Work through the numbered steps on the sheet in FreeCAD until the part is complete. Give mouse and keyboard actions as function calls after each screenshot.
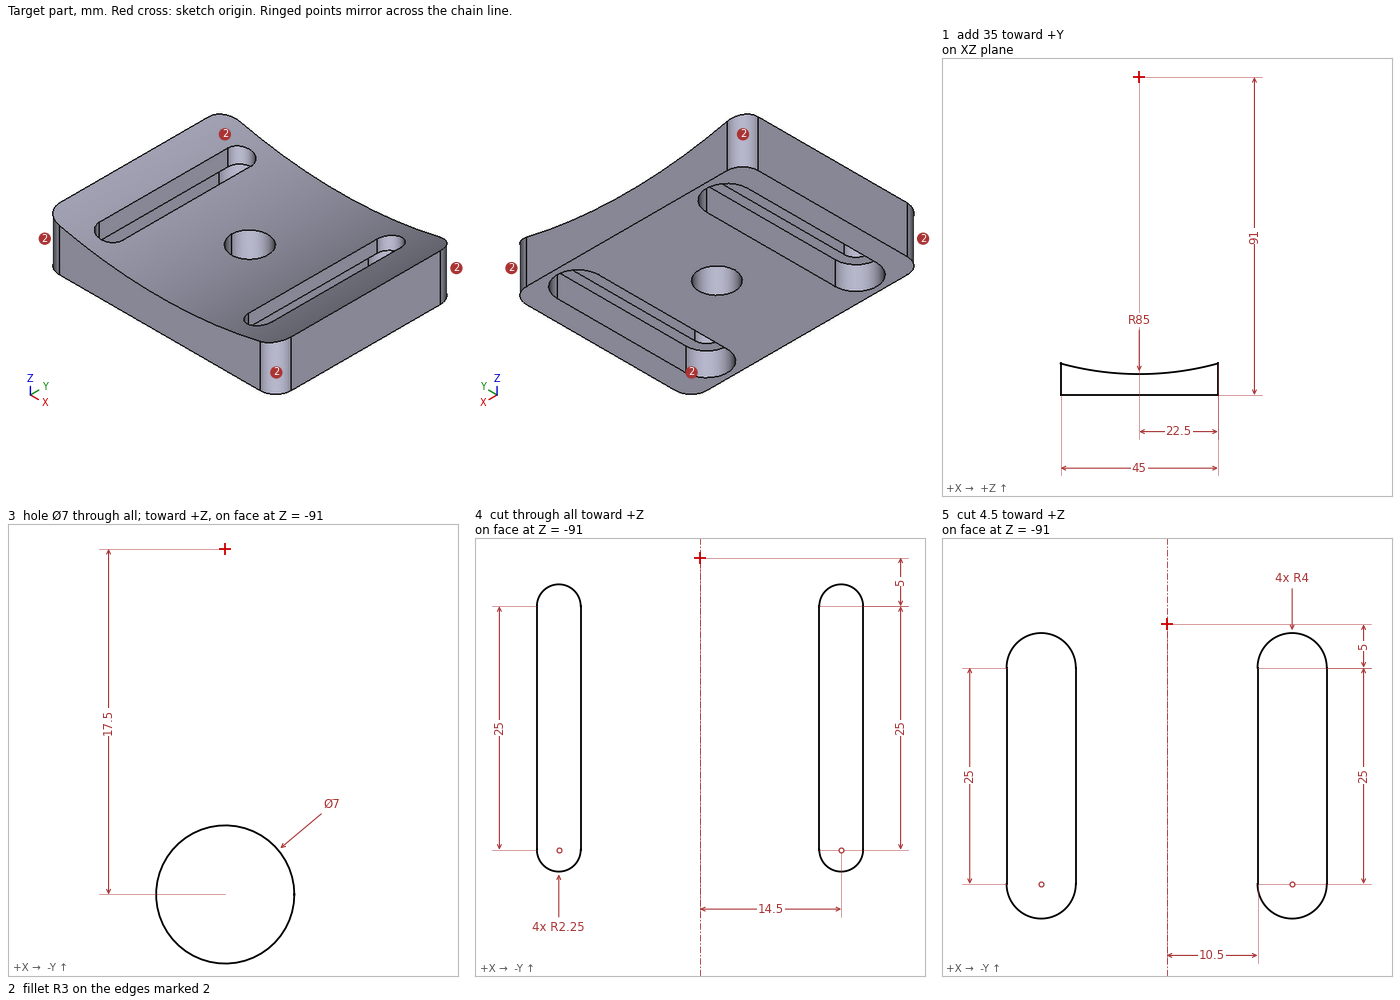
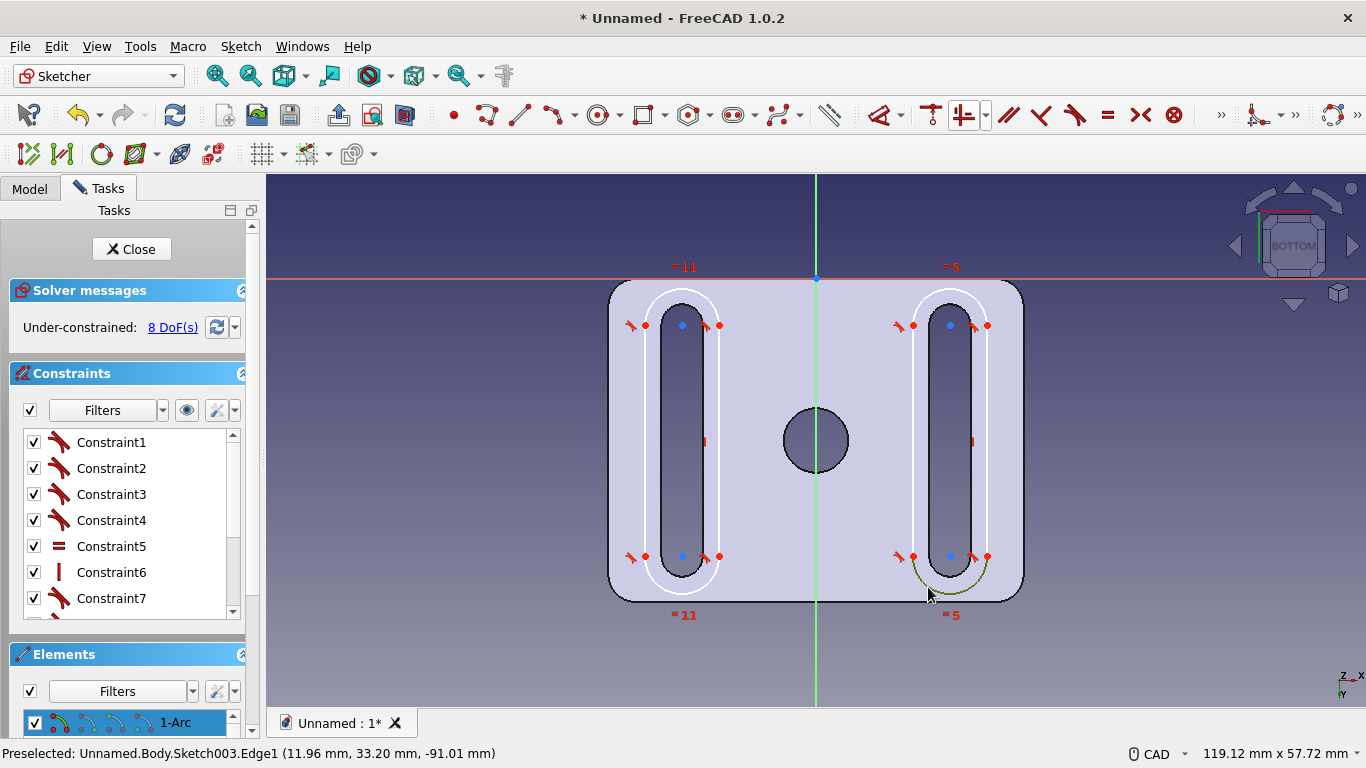
click(660, 587)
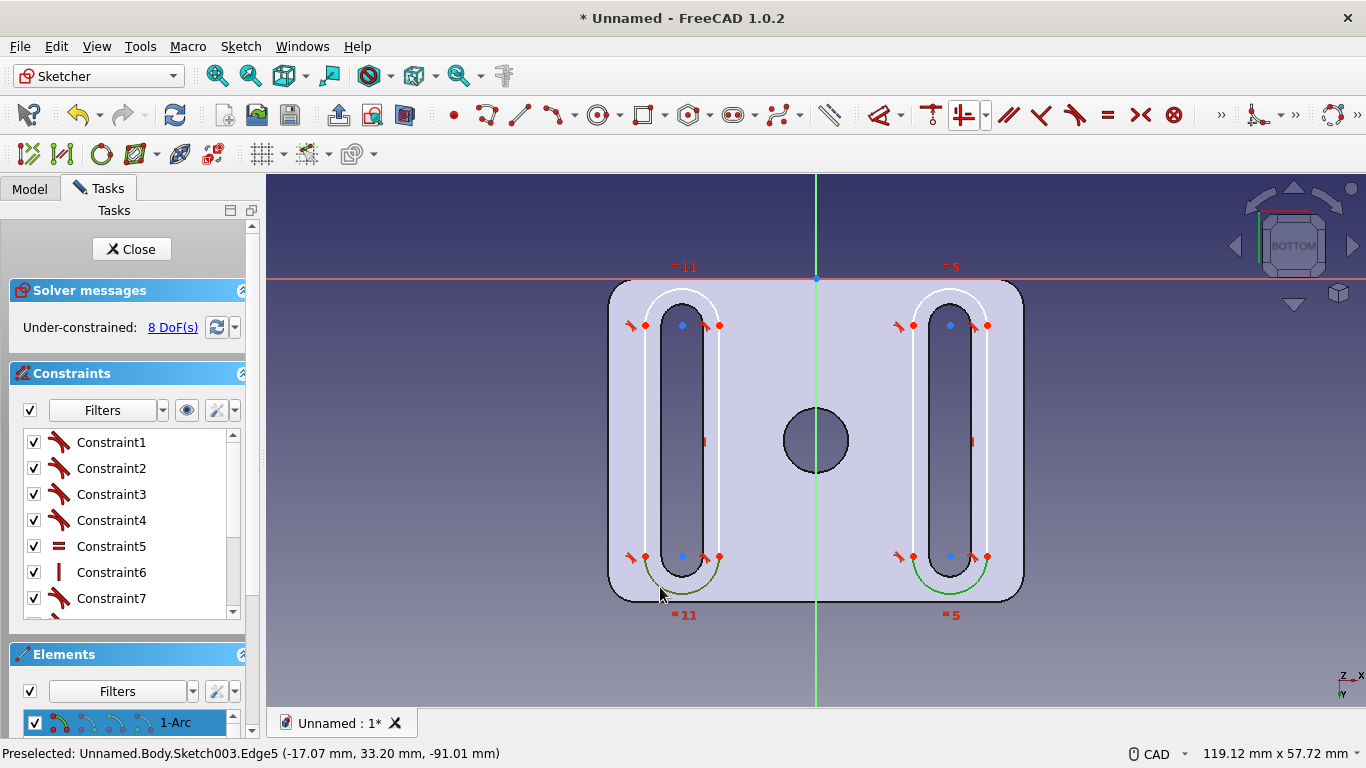
key(e)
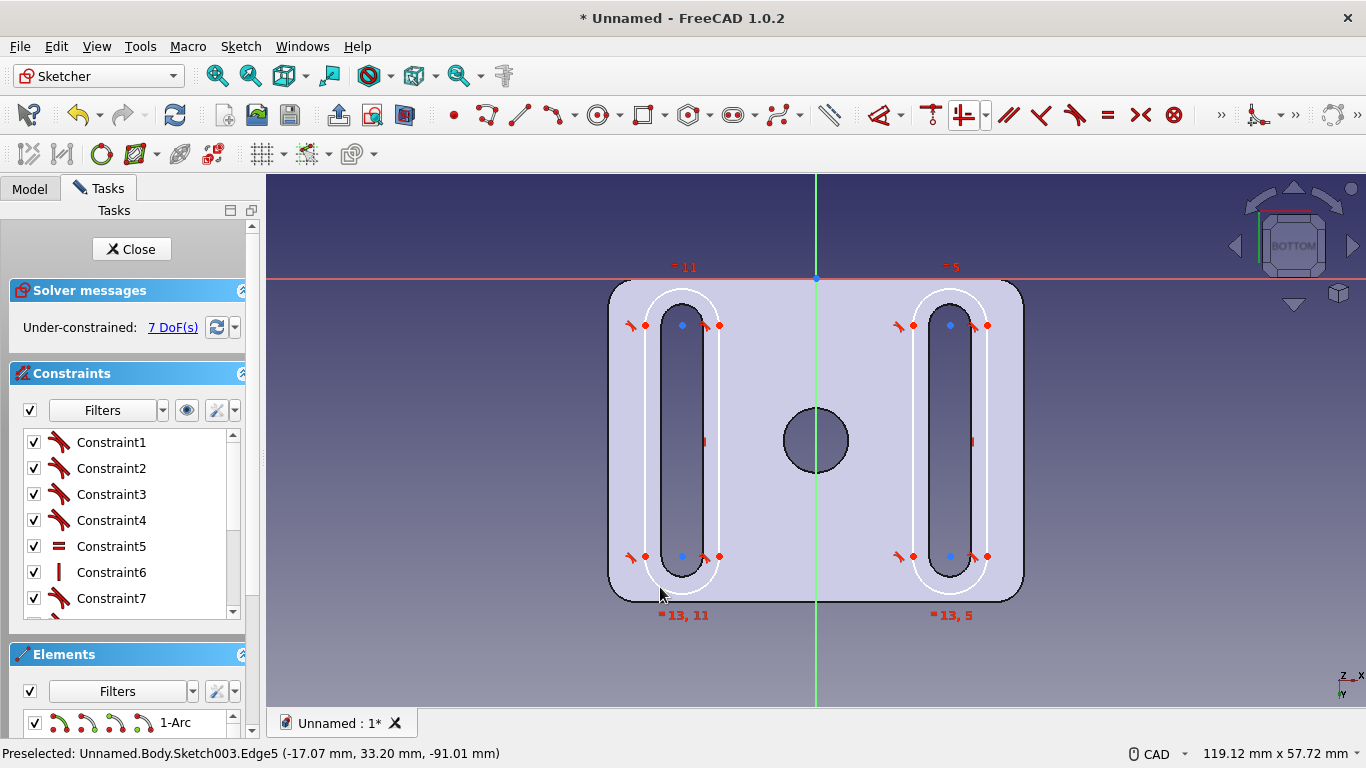
click(950, 557)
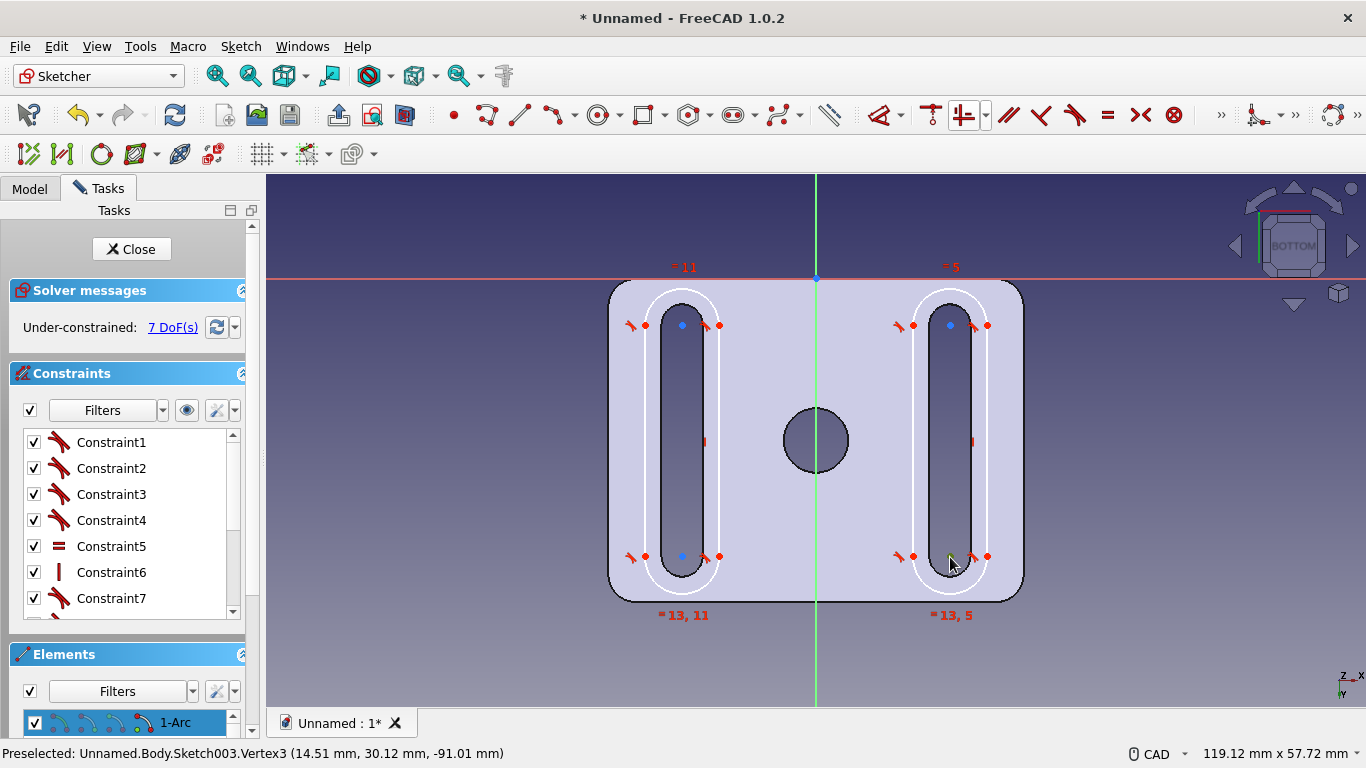
click(682, 557)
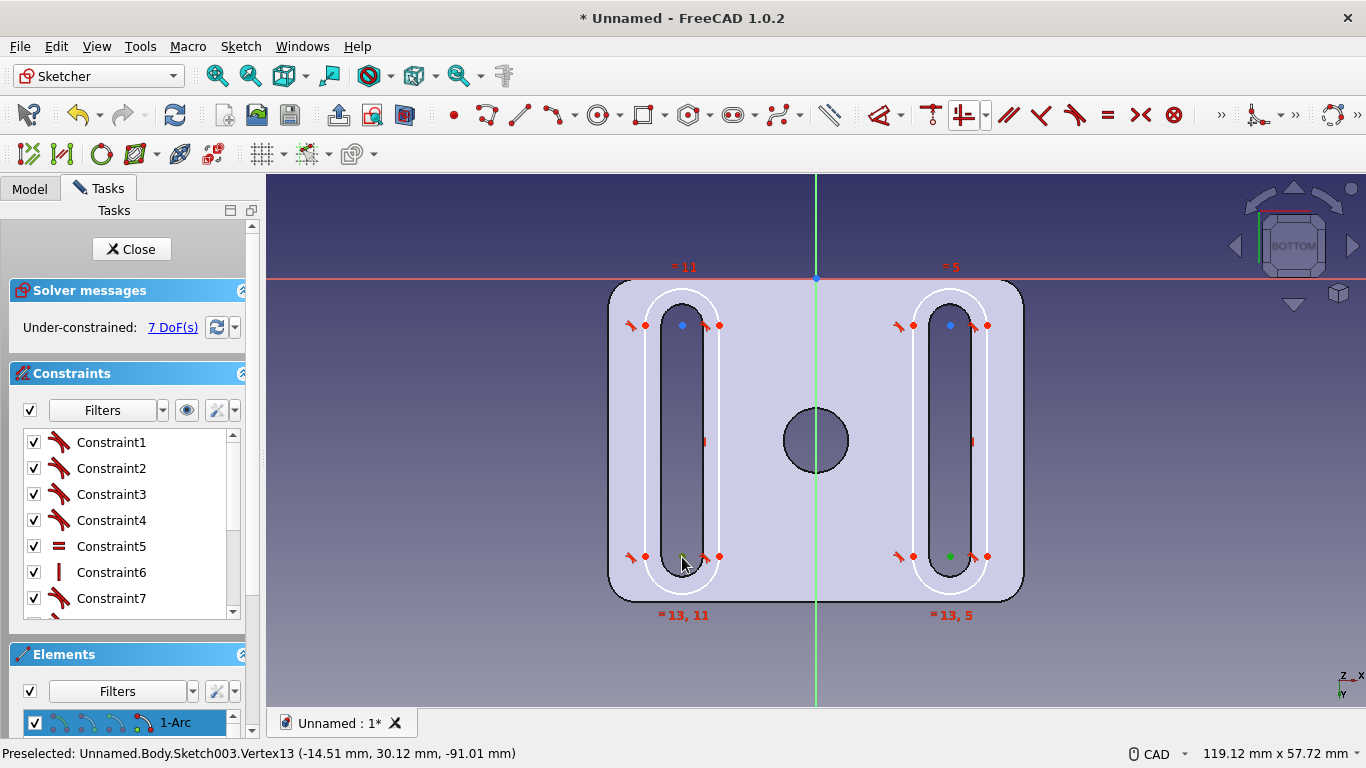
click(816, 645)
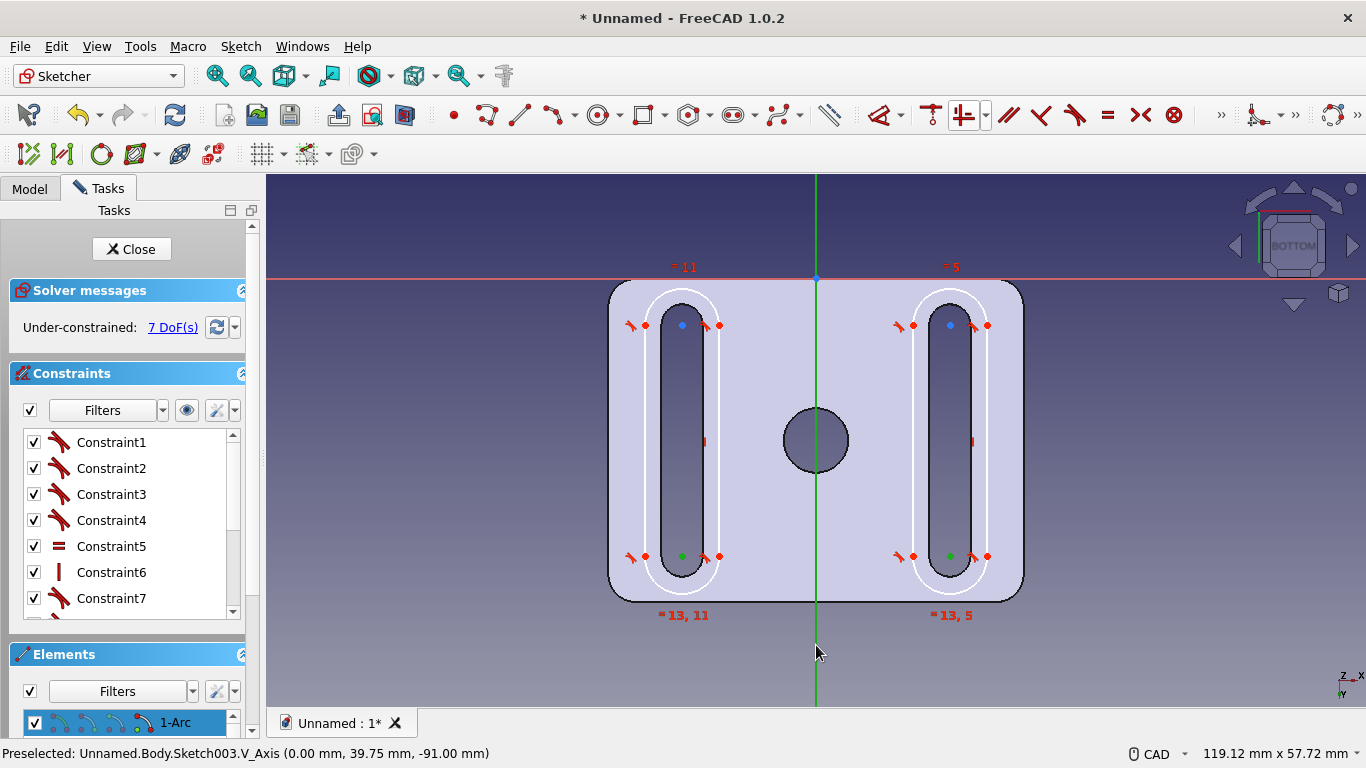
key(s)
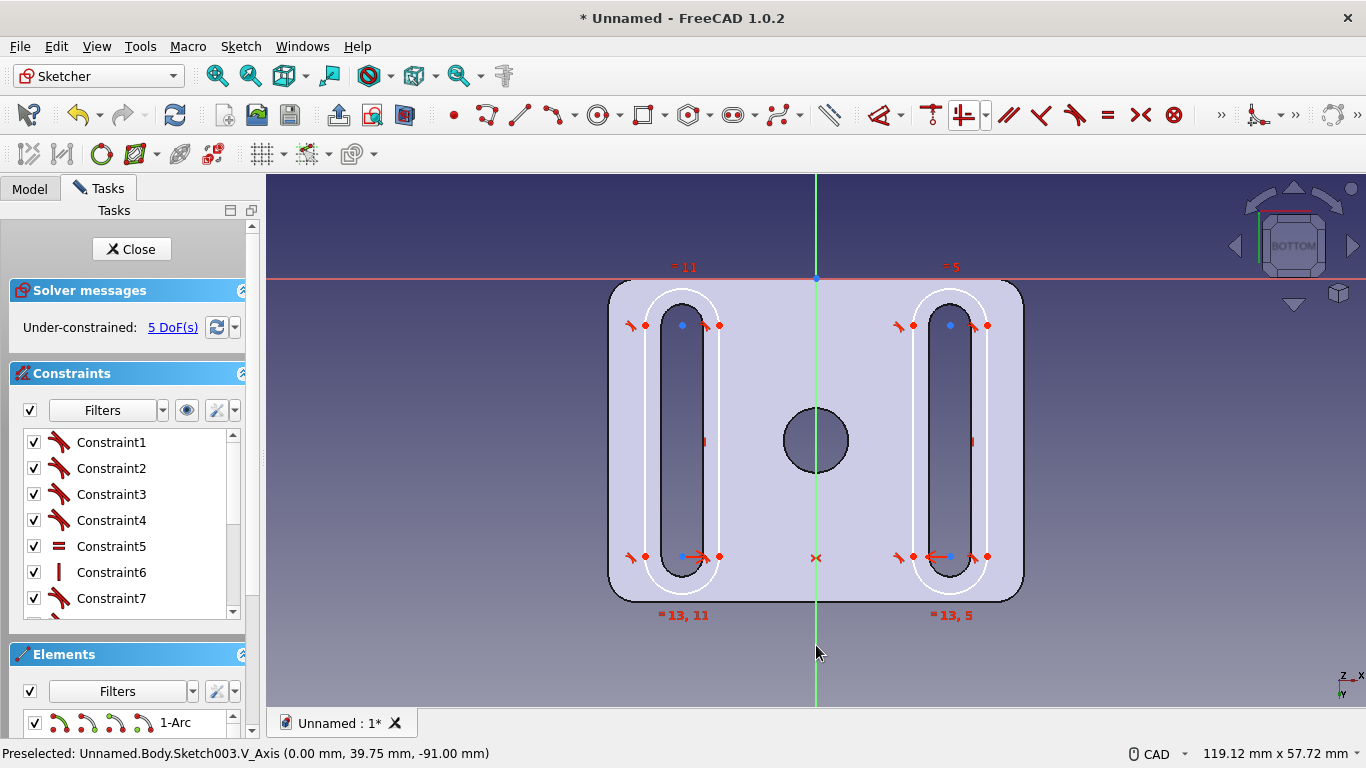
key(d)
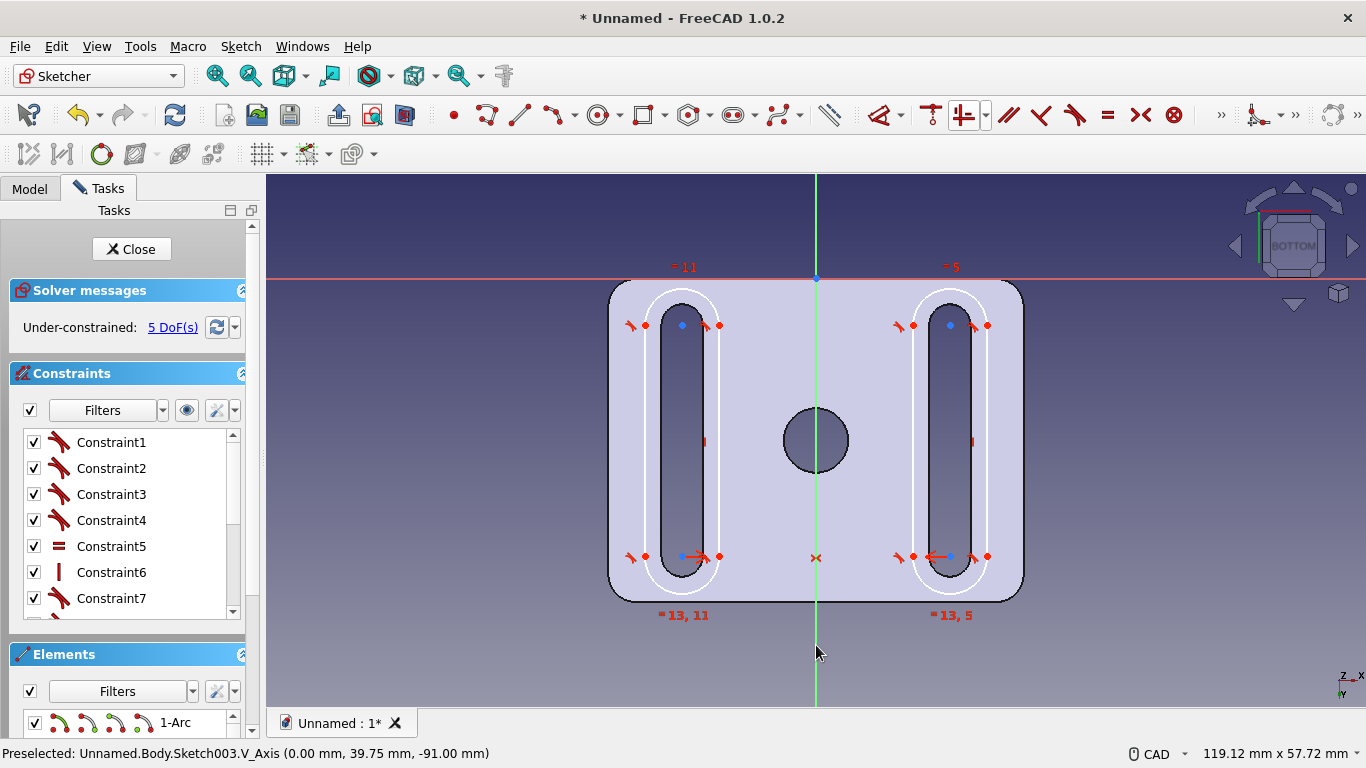
click(928, 587)
click(909, 613)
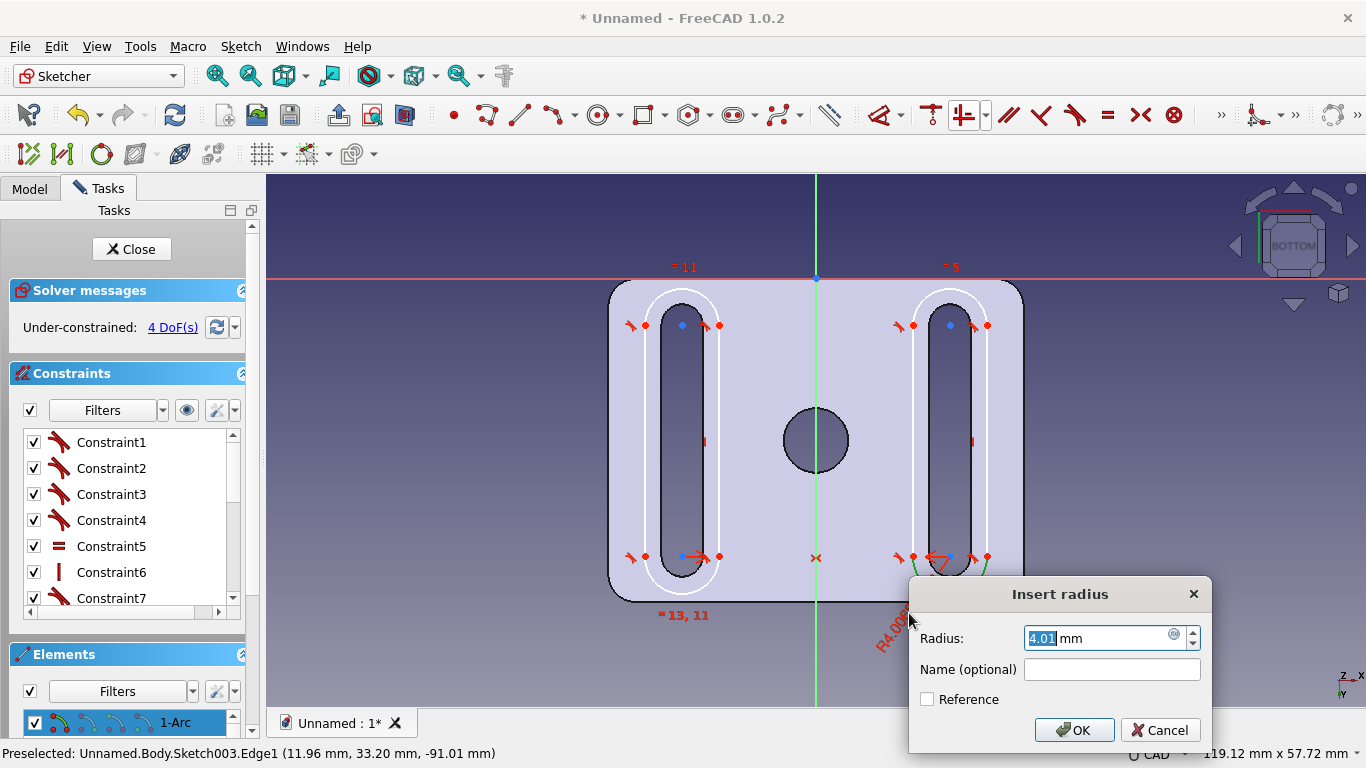
text(4)
key(Return)